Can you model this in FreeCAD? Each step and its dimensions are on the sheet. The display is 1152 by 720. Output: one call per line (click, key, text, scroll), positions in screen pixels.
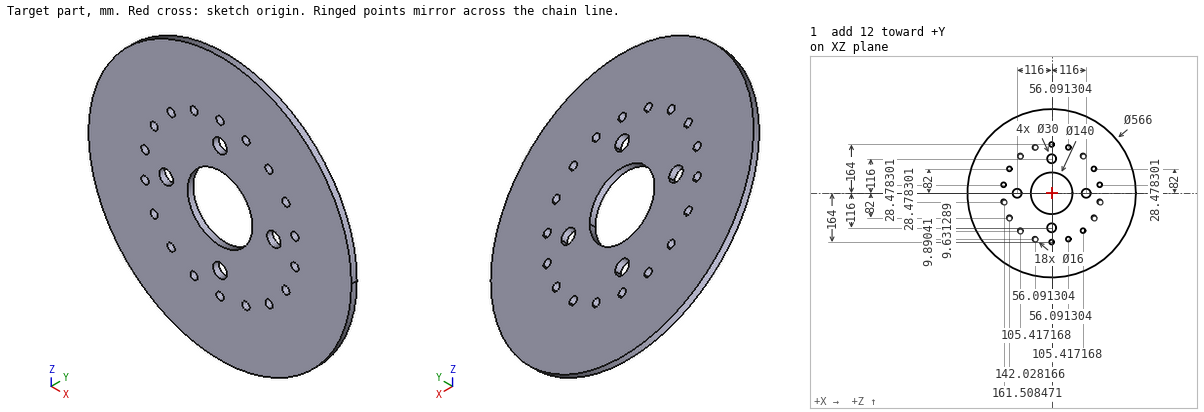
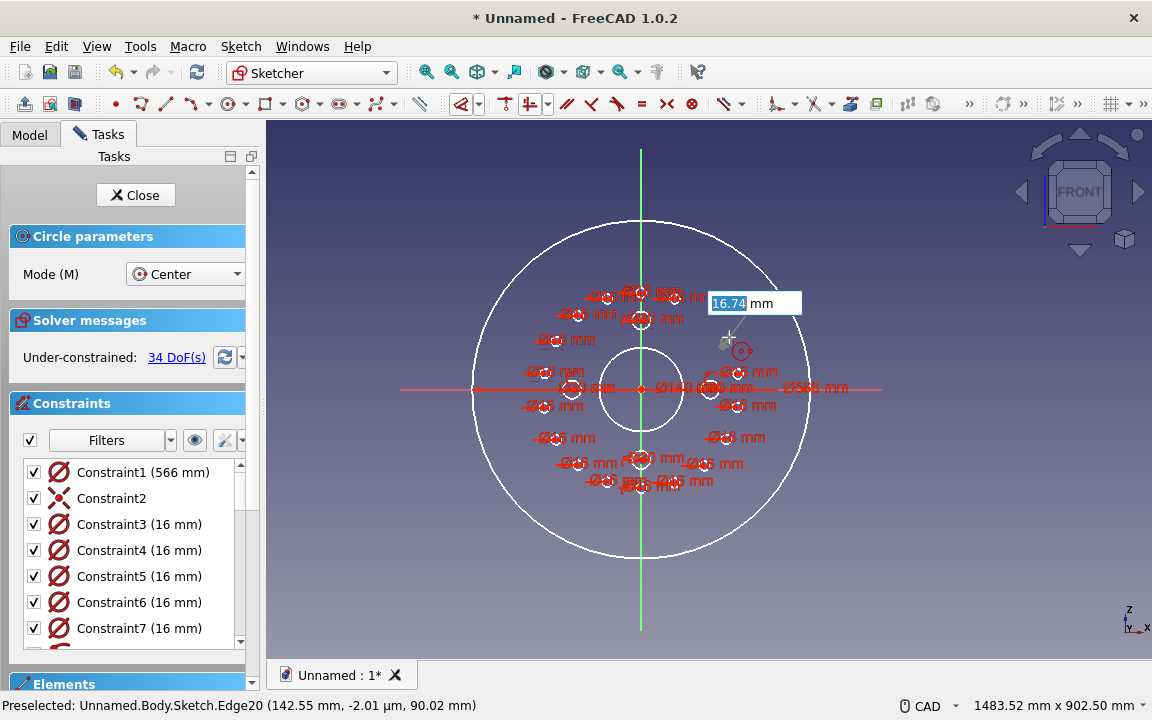
text(16)
key(Return)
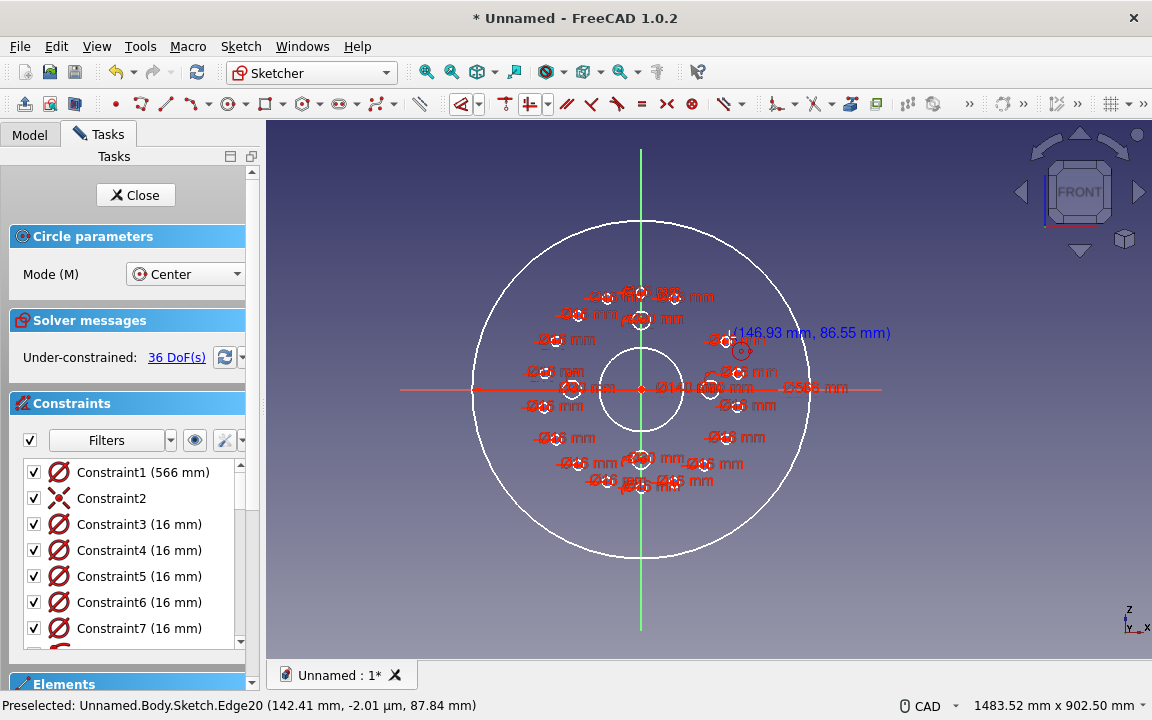
scroll(704, 315, up, 8)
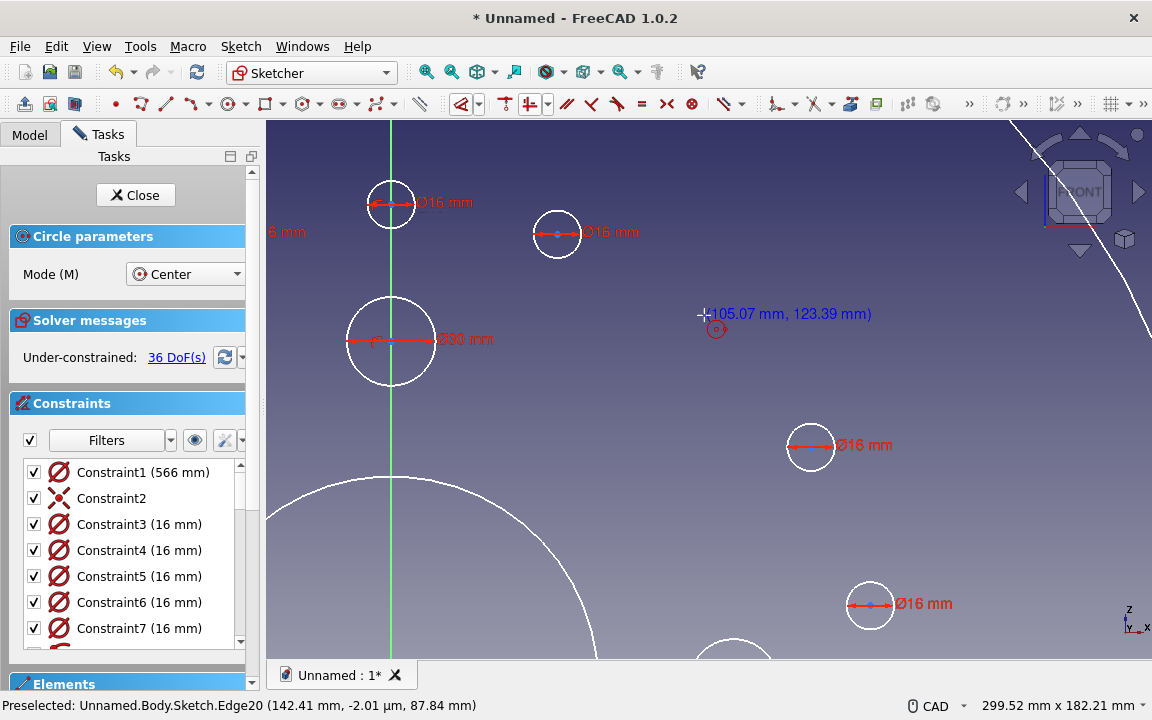
scroll(704, 315, down, 8)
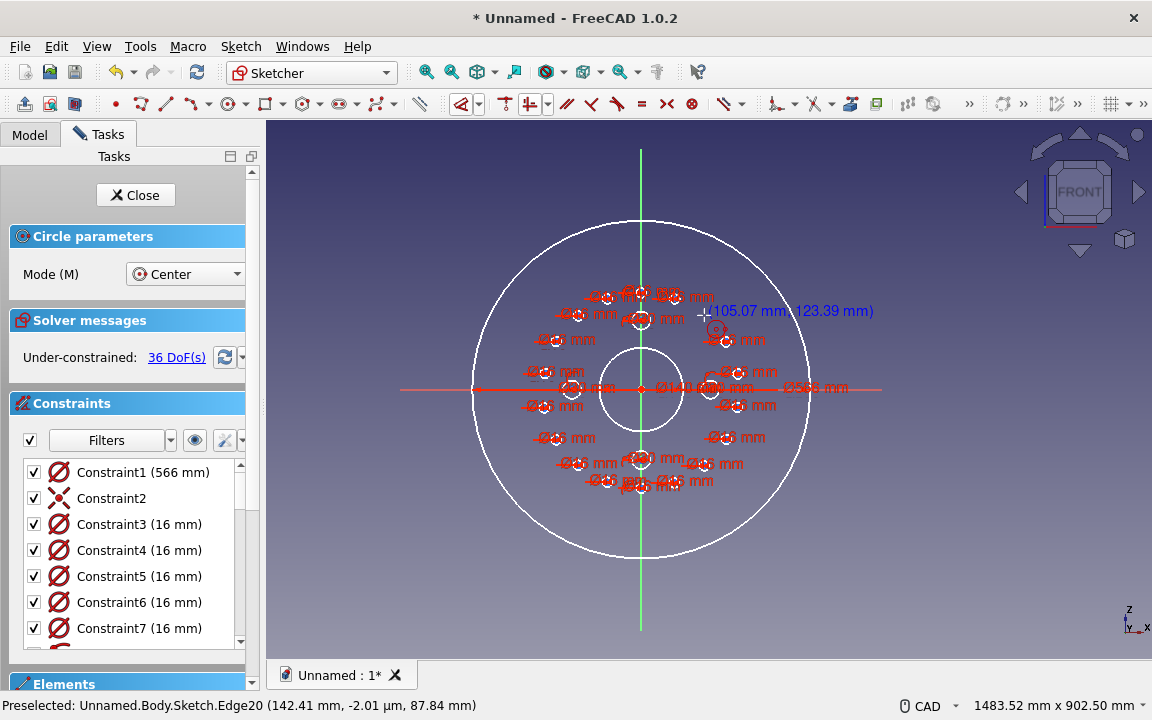
click(704, 315)
move(708, 311)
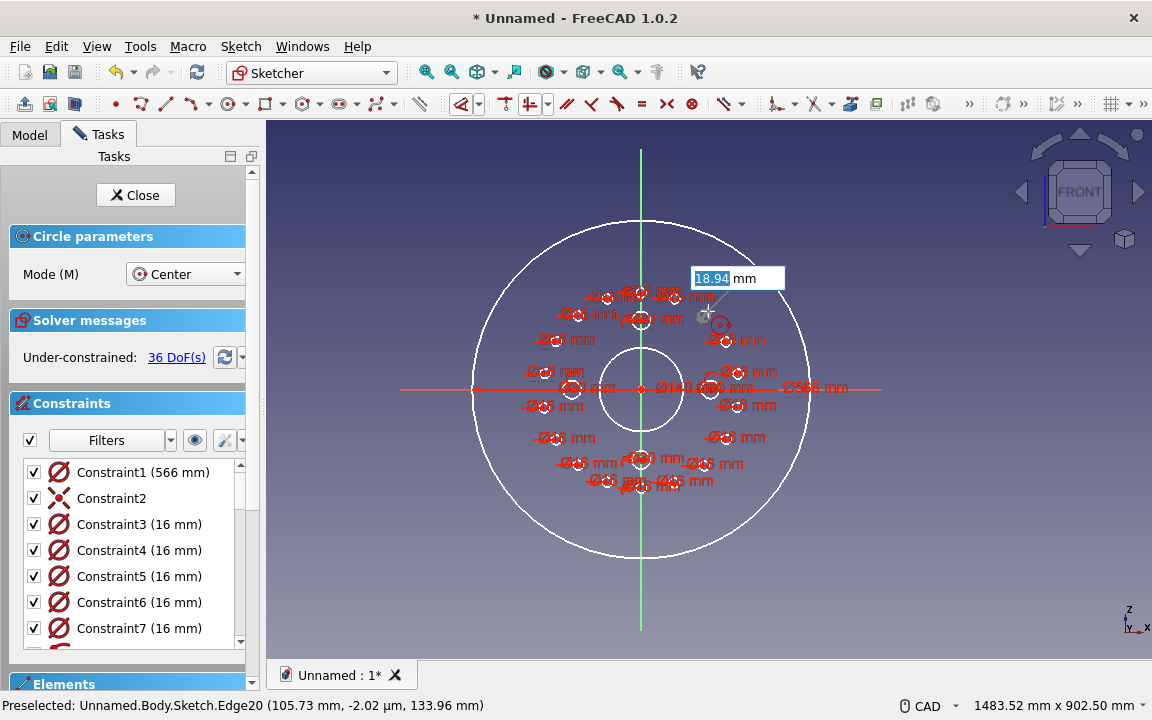
text(16)
key(Return)
key(Escape)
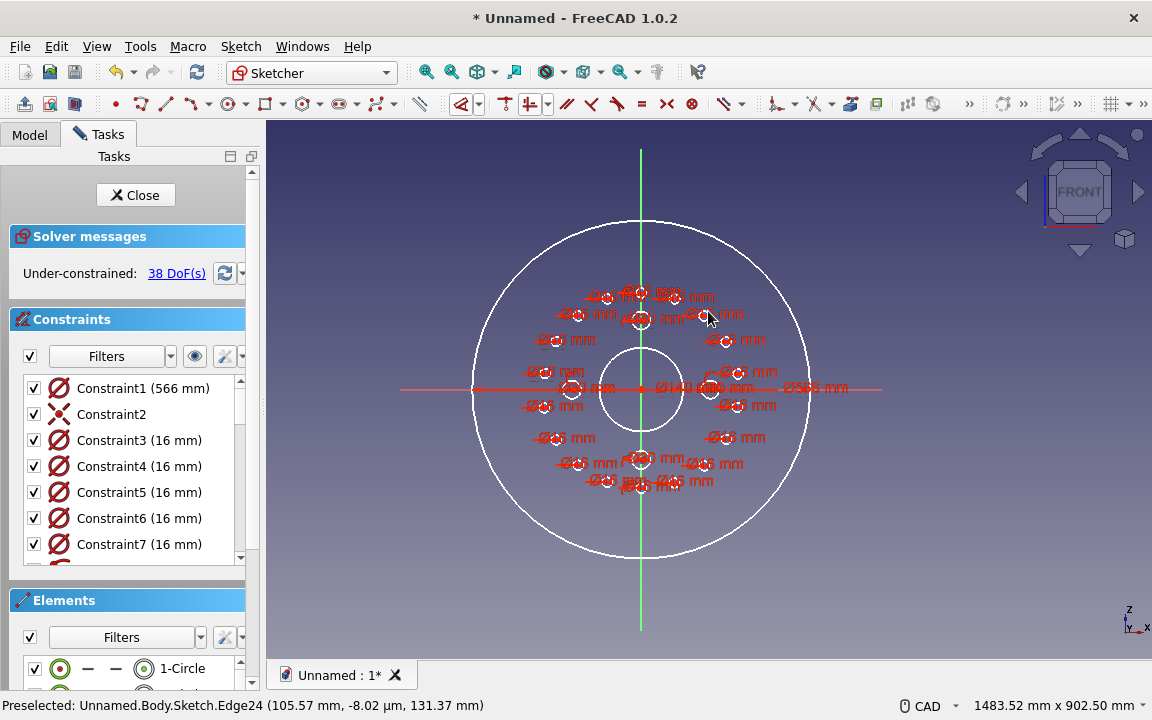
click(544, 408)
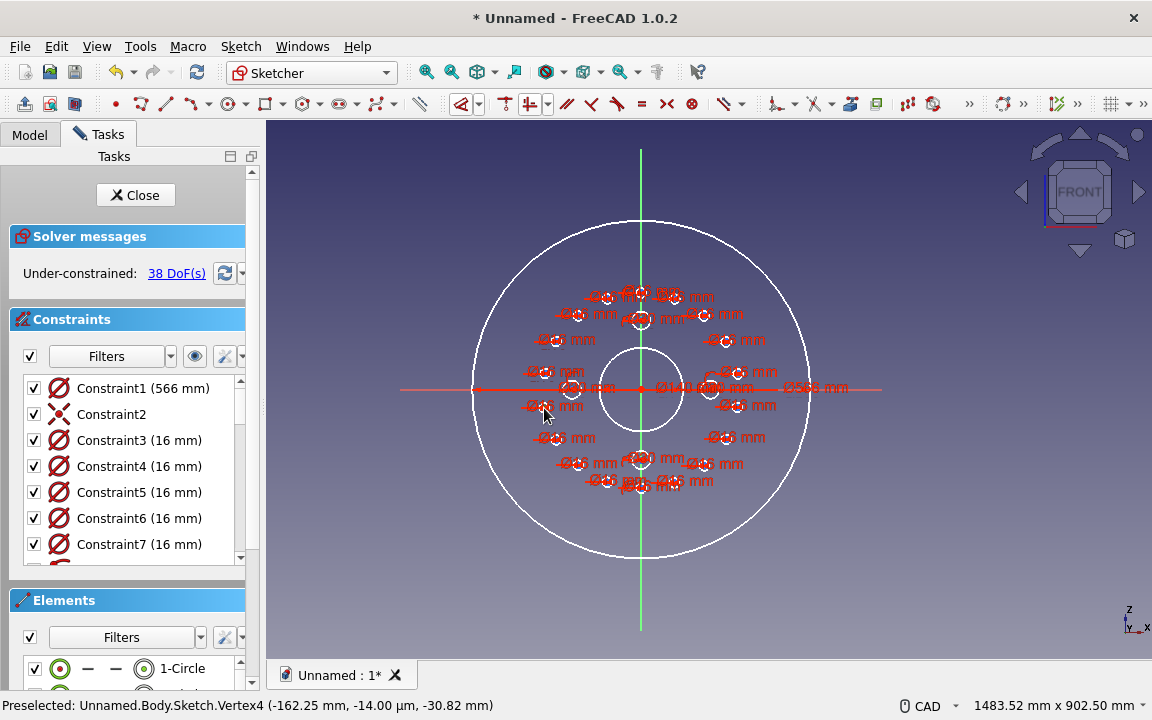
click(545, 374)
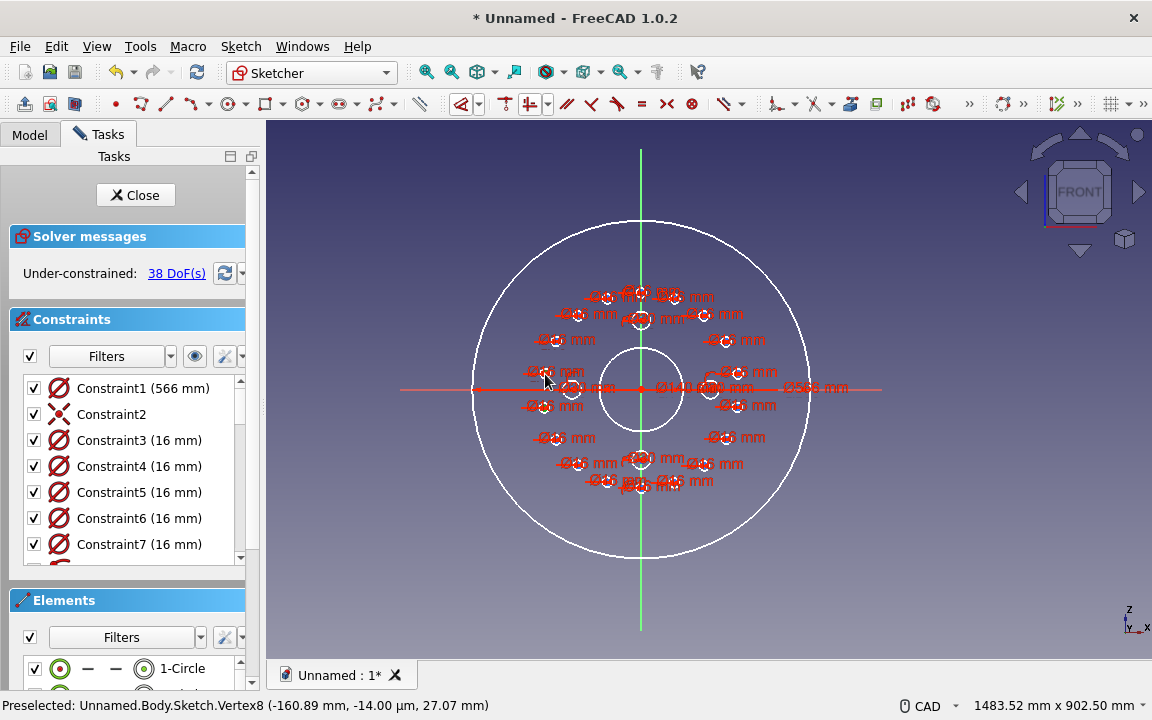
key(v)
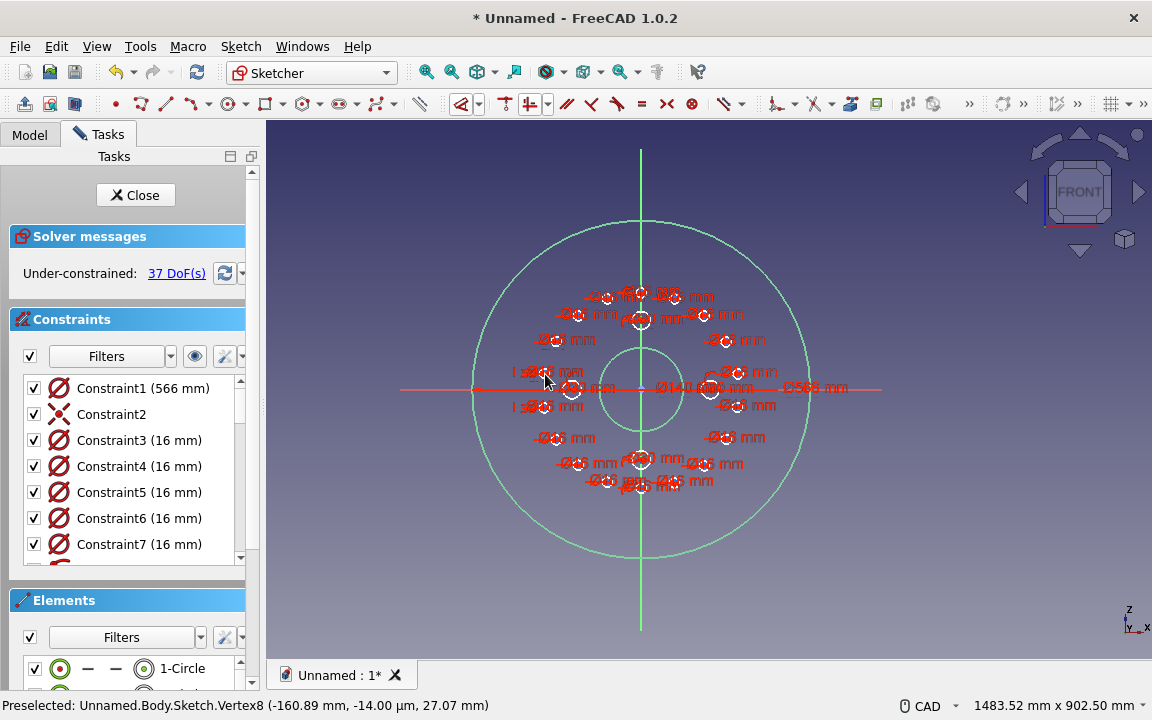
click(556, 440)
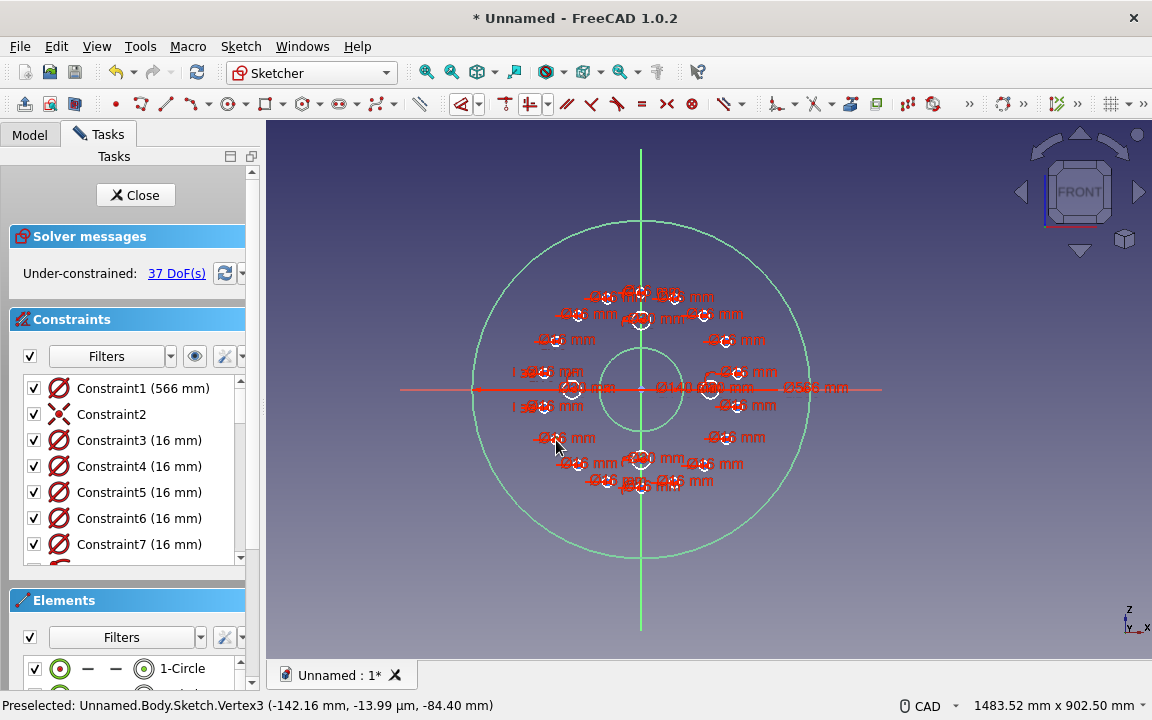
click(556, 342)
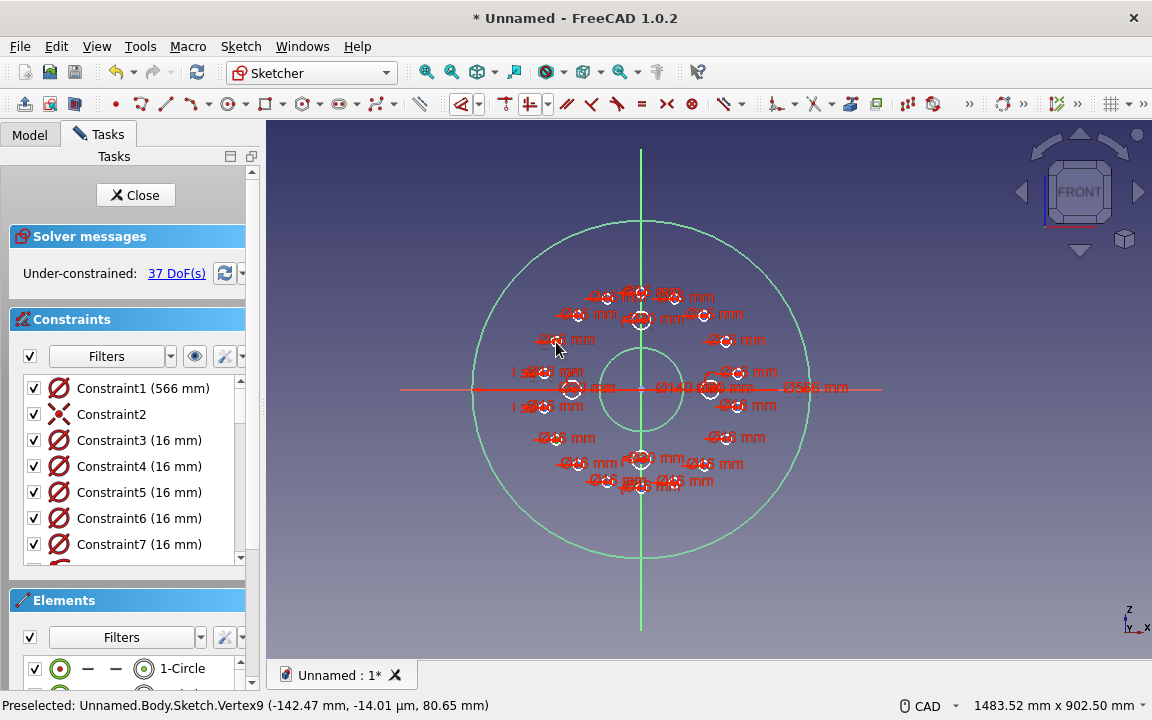
key(v)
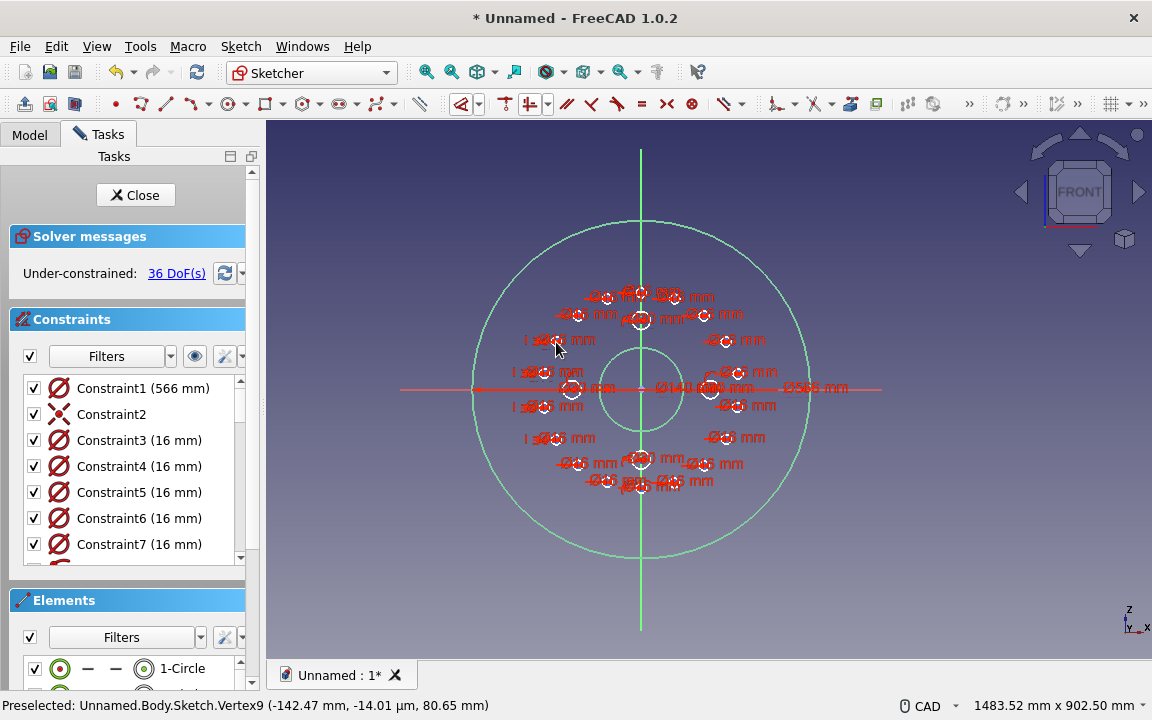
click(607, 482)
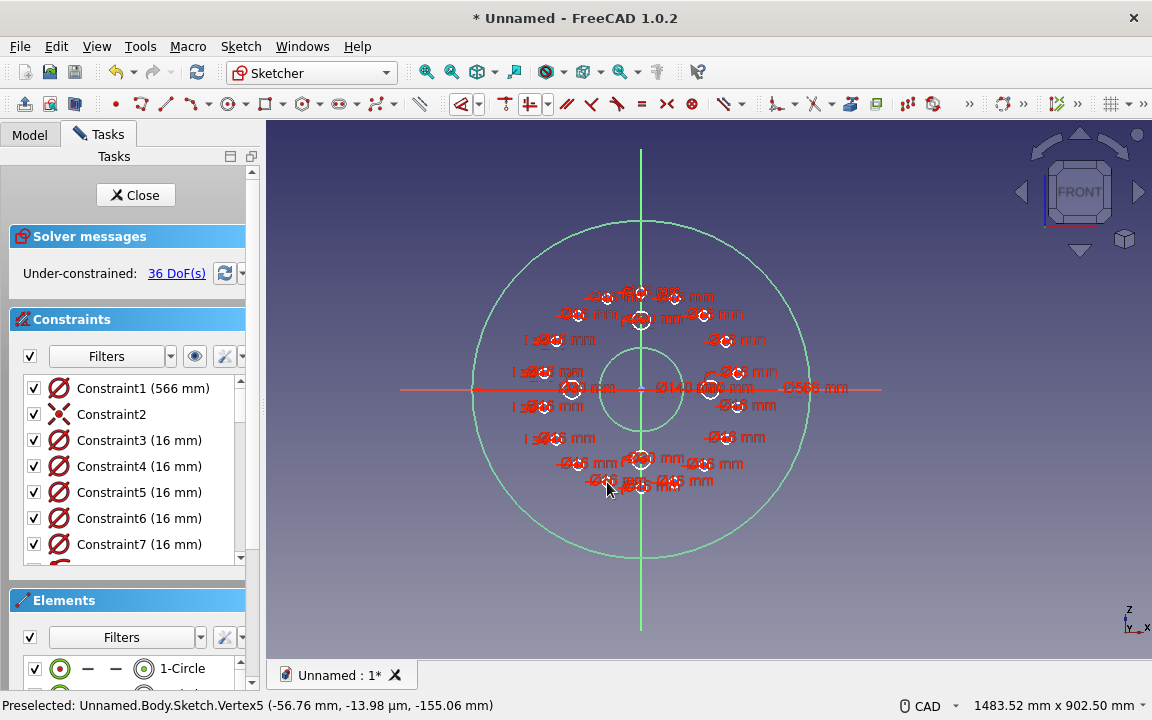
click(674, 483)